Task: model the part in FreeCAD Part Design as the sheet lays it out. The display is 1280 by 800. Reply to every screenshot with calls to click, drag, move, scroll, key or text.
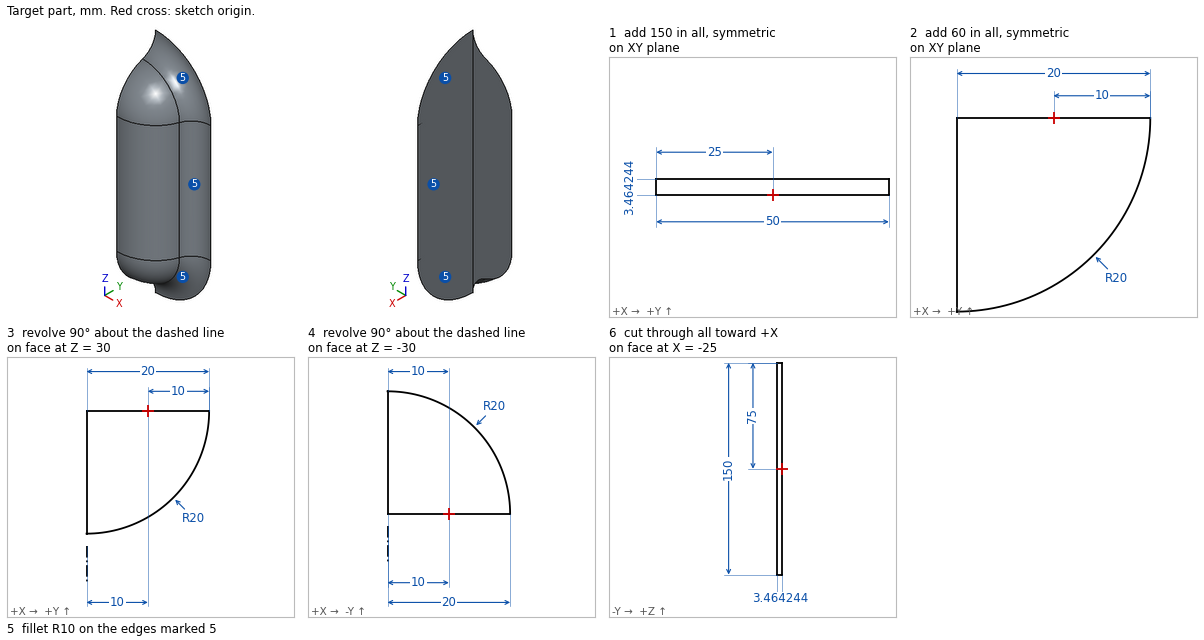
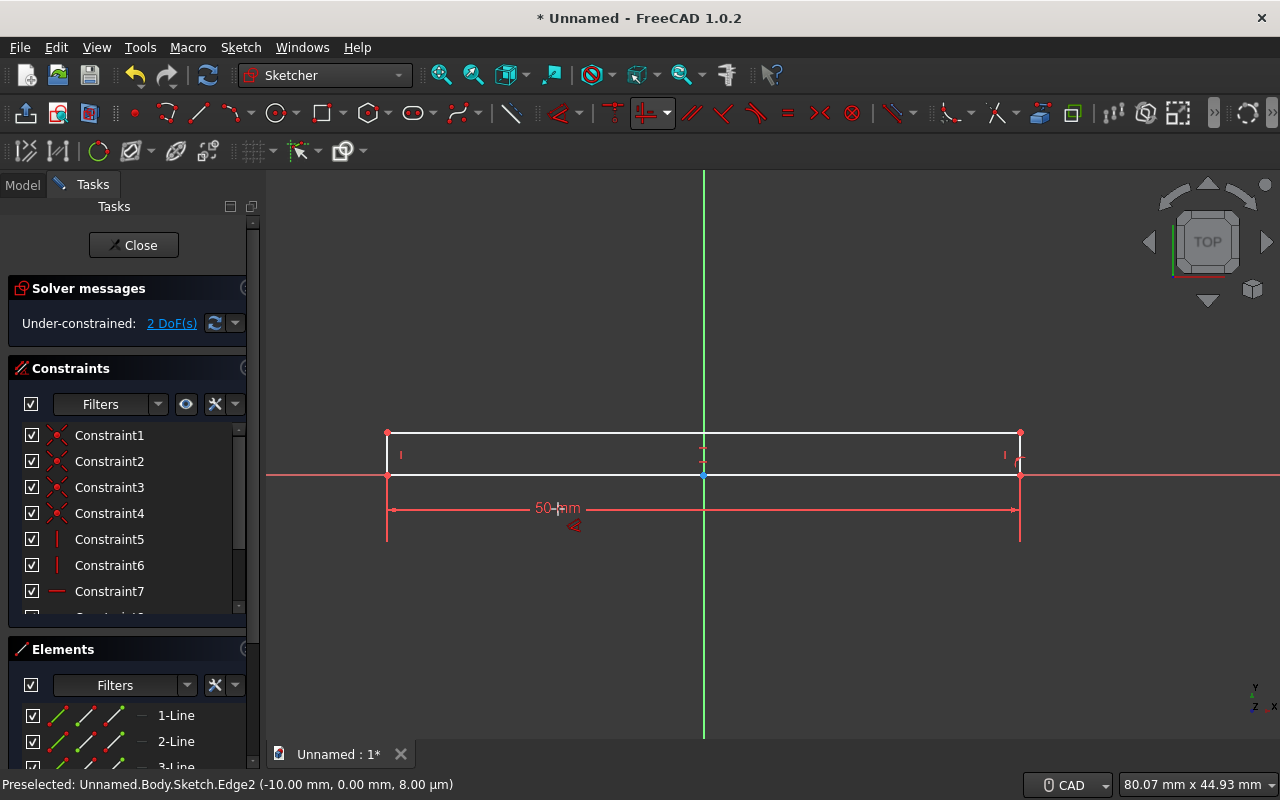
click(387, 433)
click(473, 509)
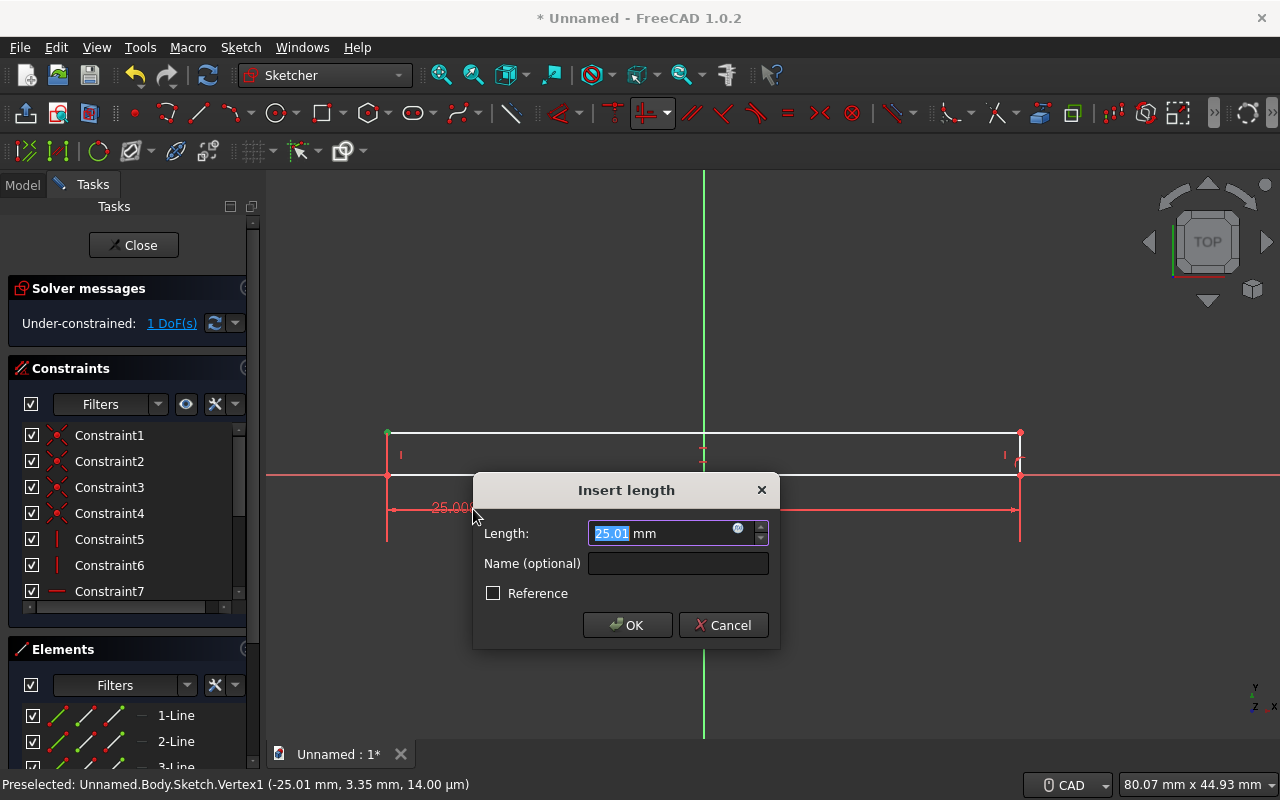
text(25)
key(Return)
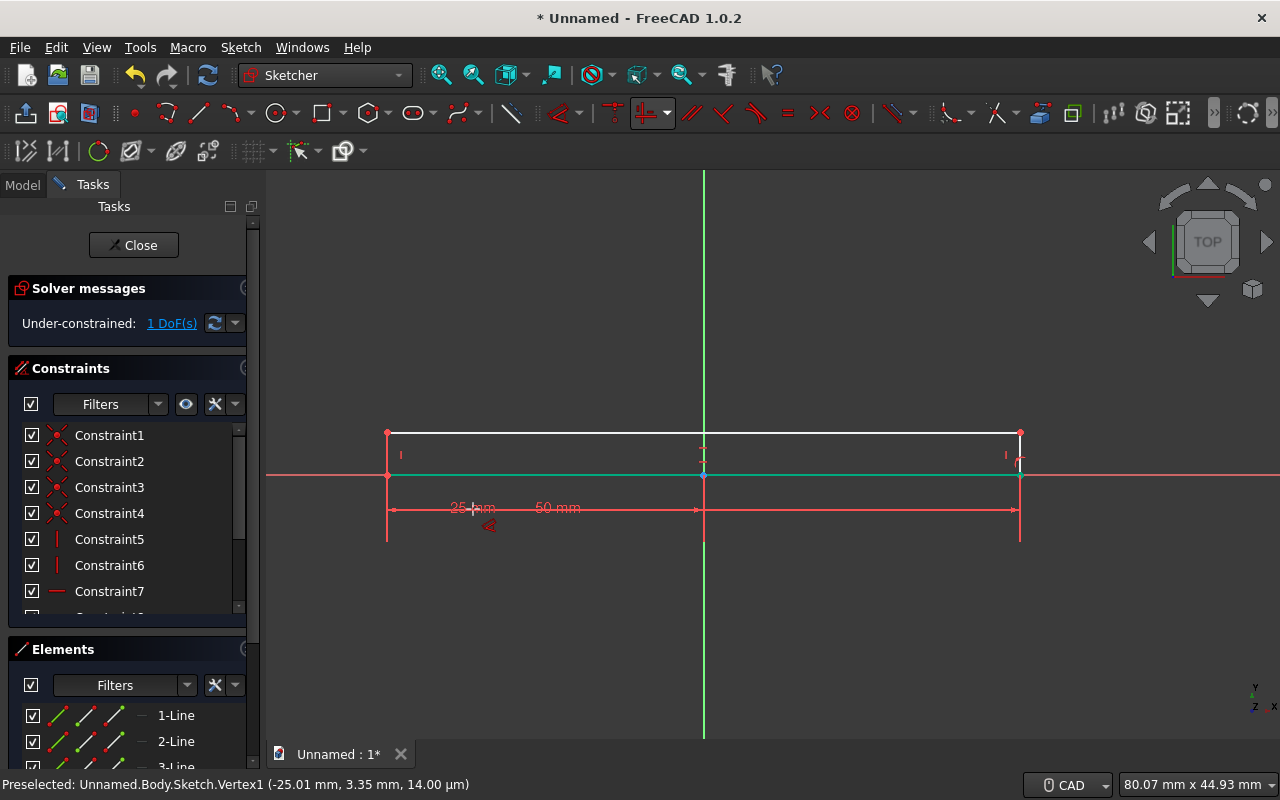
click(387, 446)
click(353, 454)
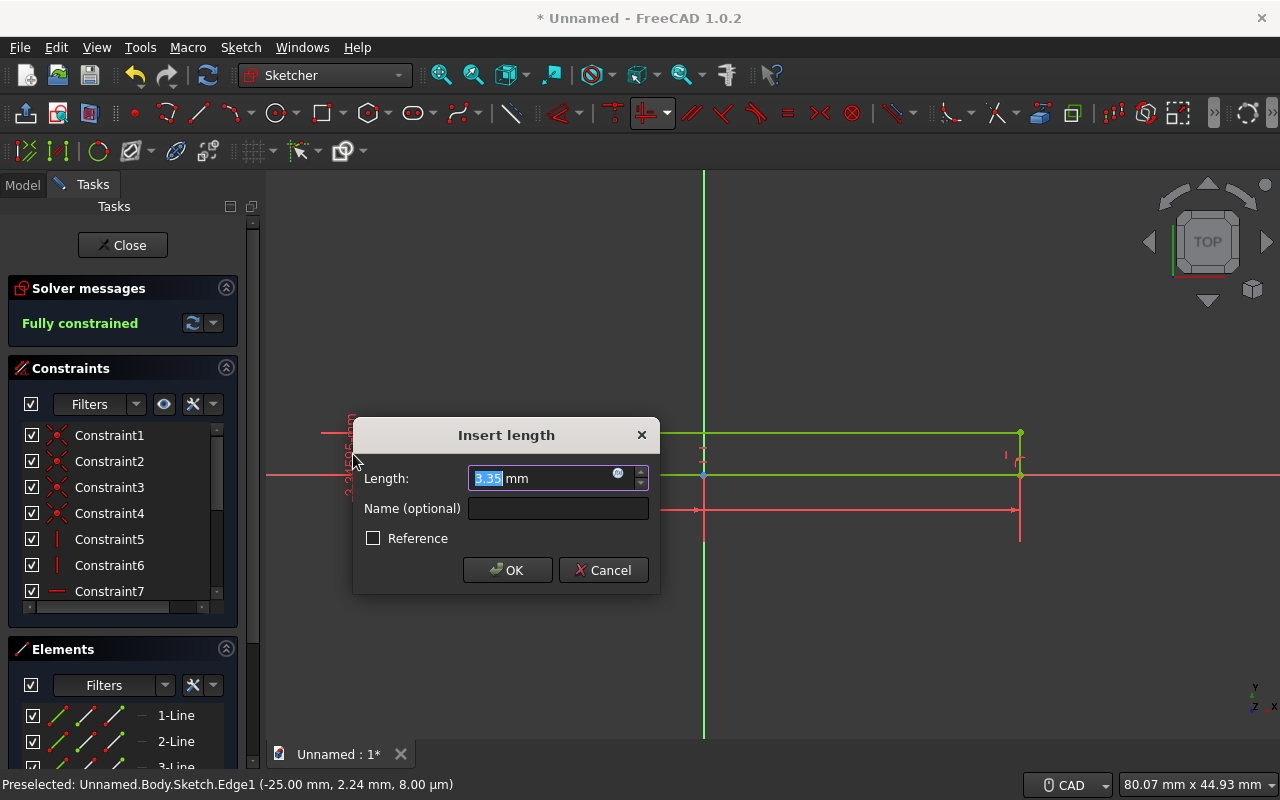
text(3.464244)
key(Return)
key(Escape)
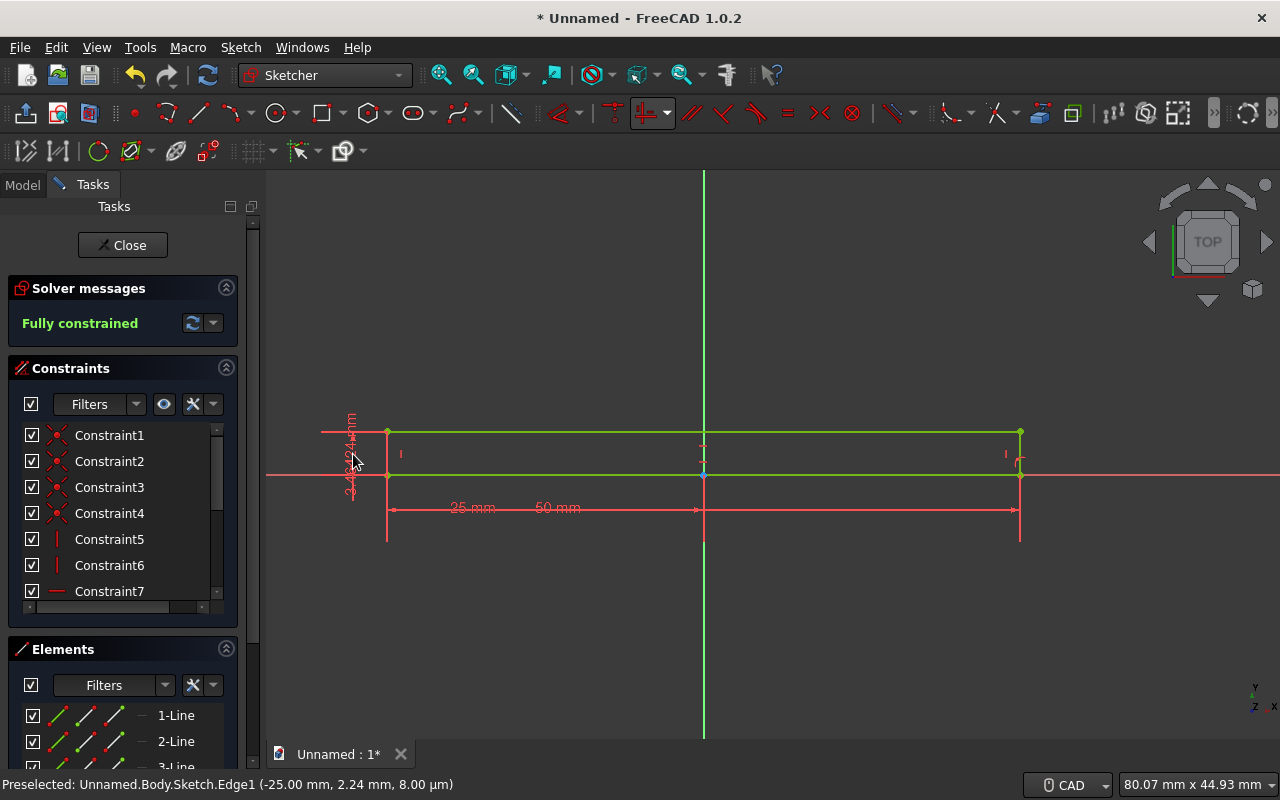
click(123, 245)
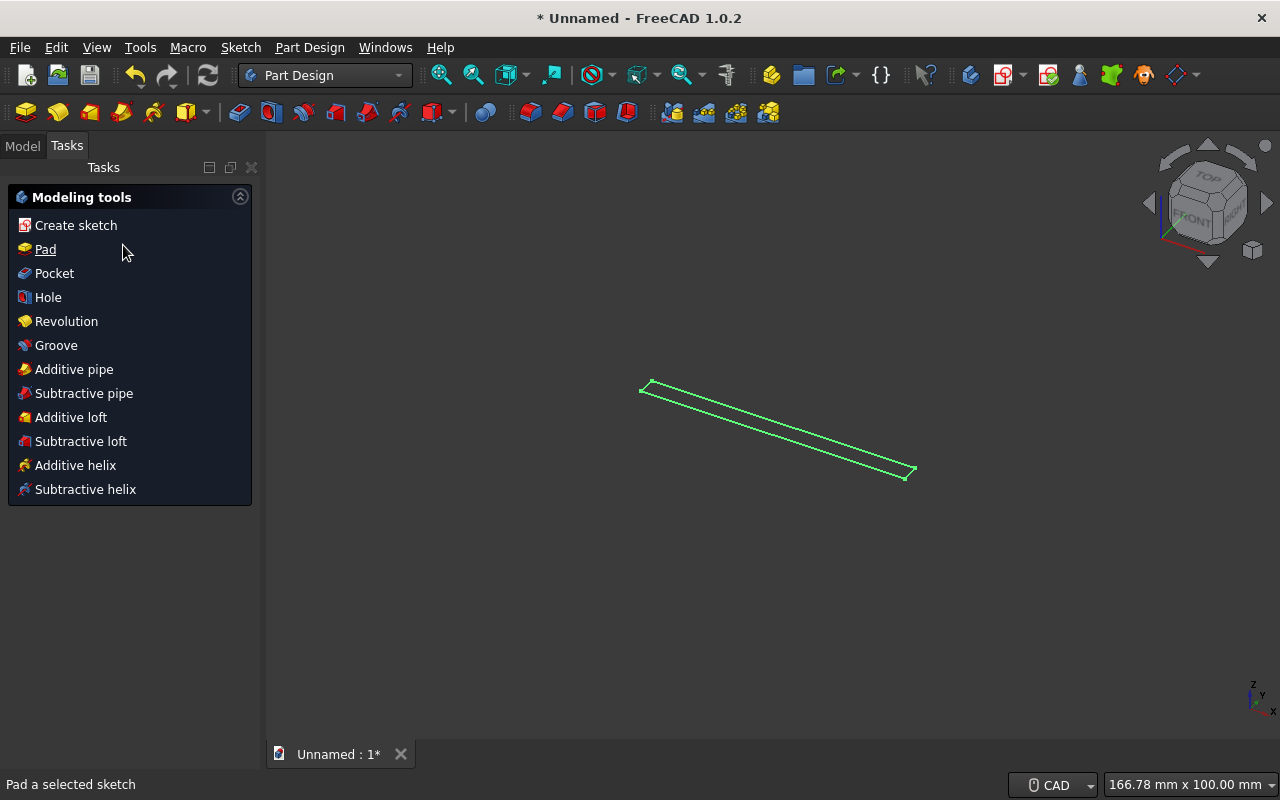
click(26, 112)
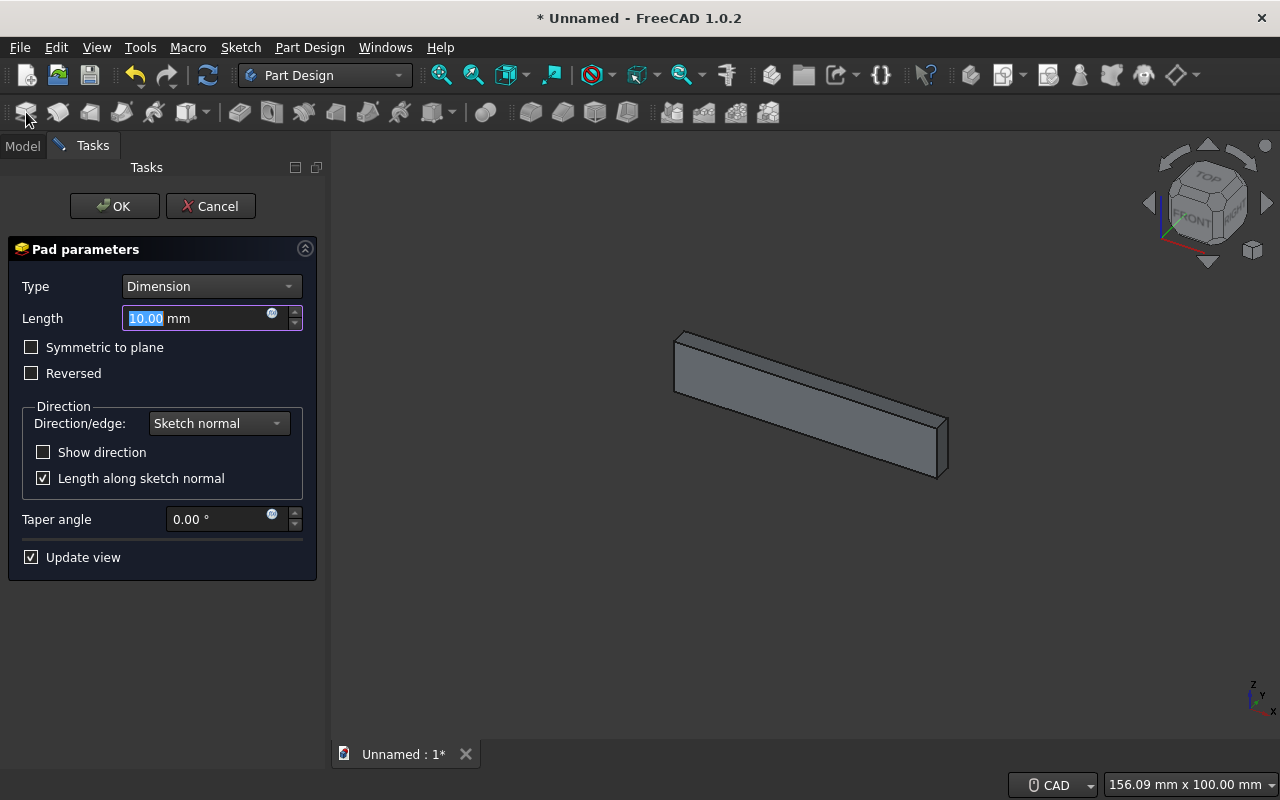
text(150)
key(Tab)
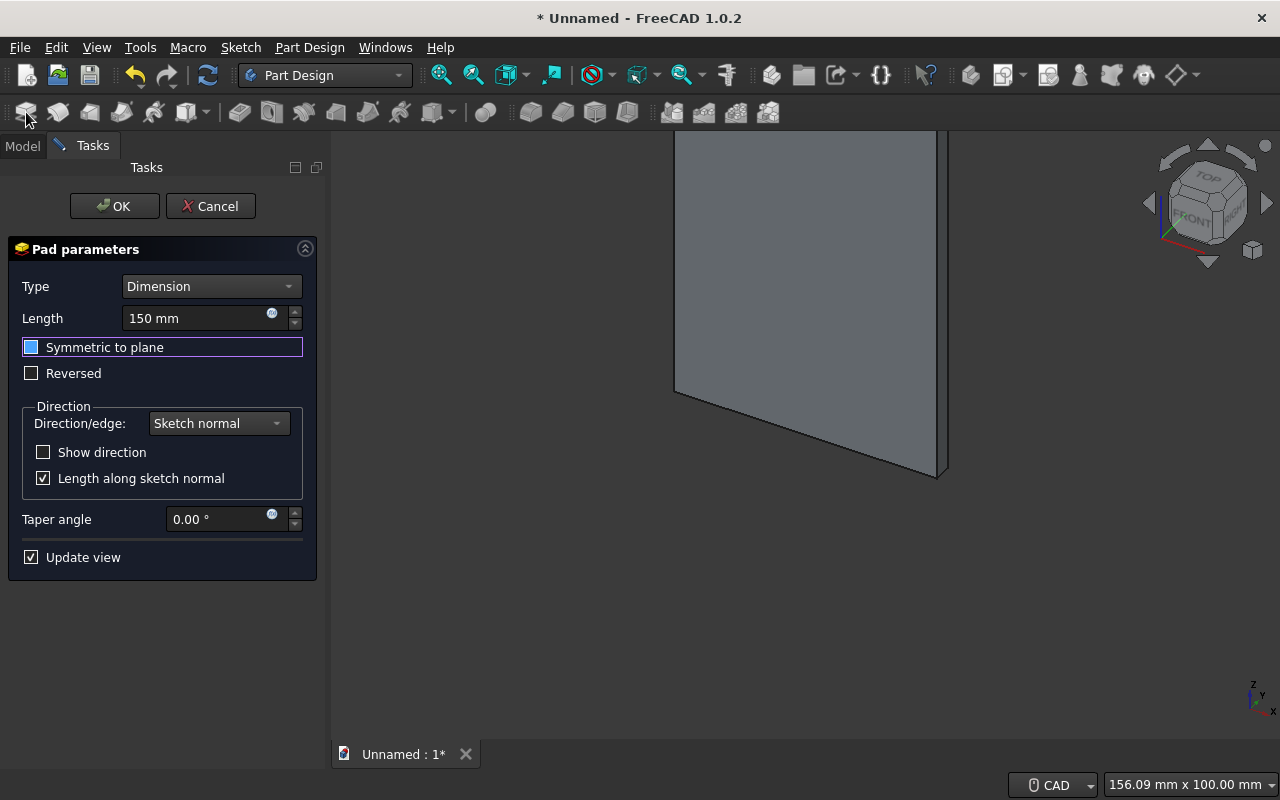
click(30, 347)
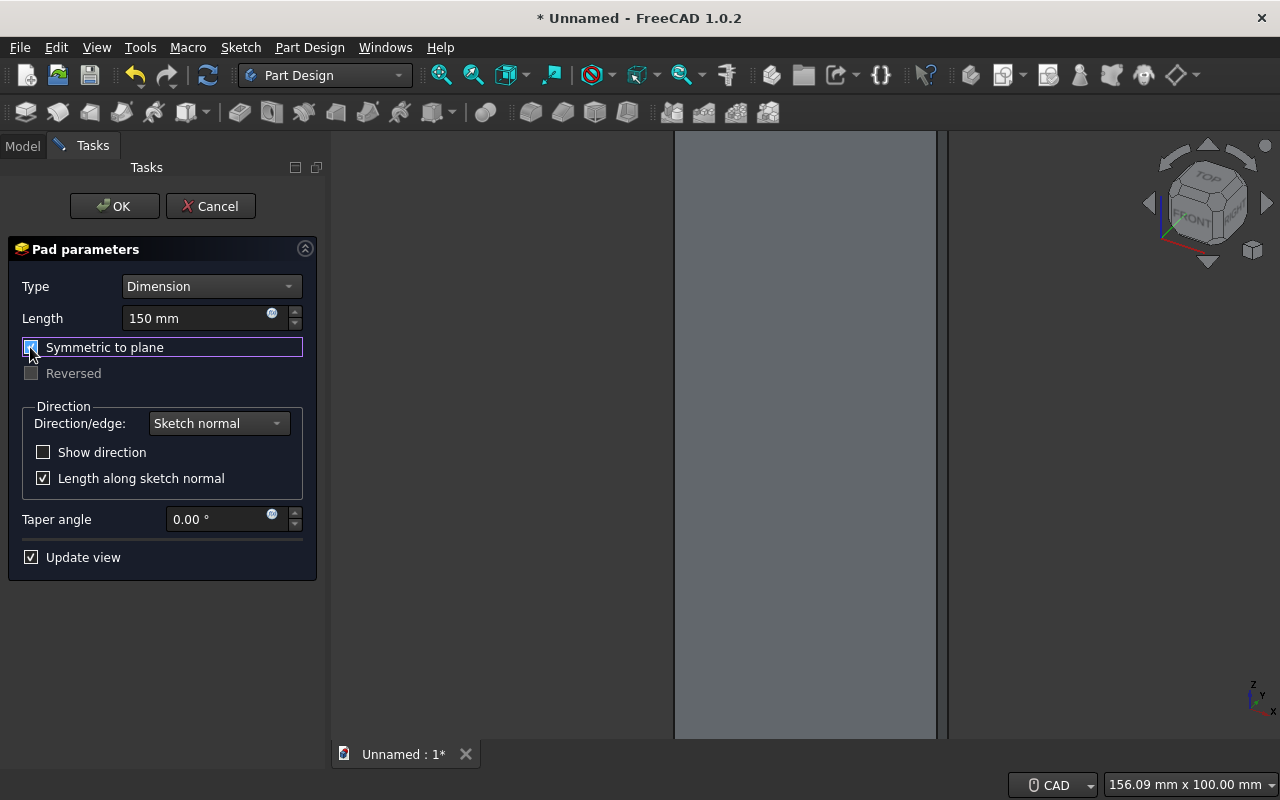
click(115, 206)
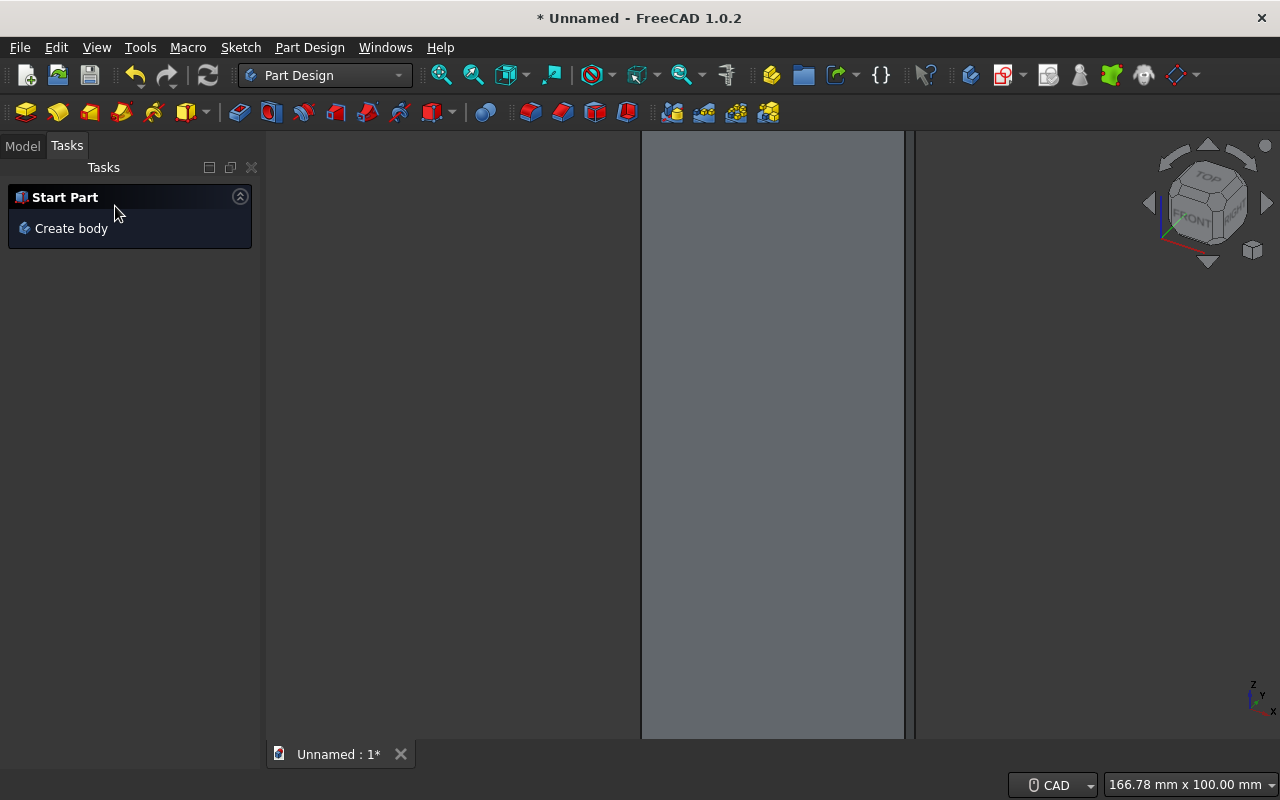
click(442, 76)